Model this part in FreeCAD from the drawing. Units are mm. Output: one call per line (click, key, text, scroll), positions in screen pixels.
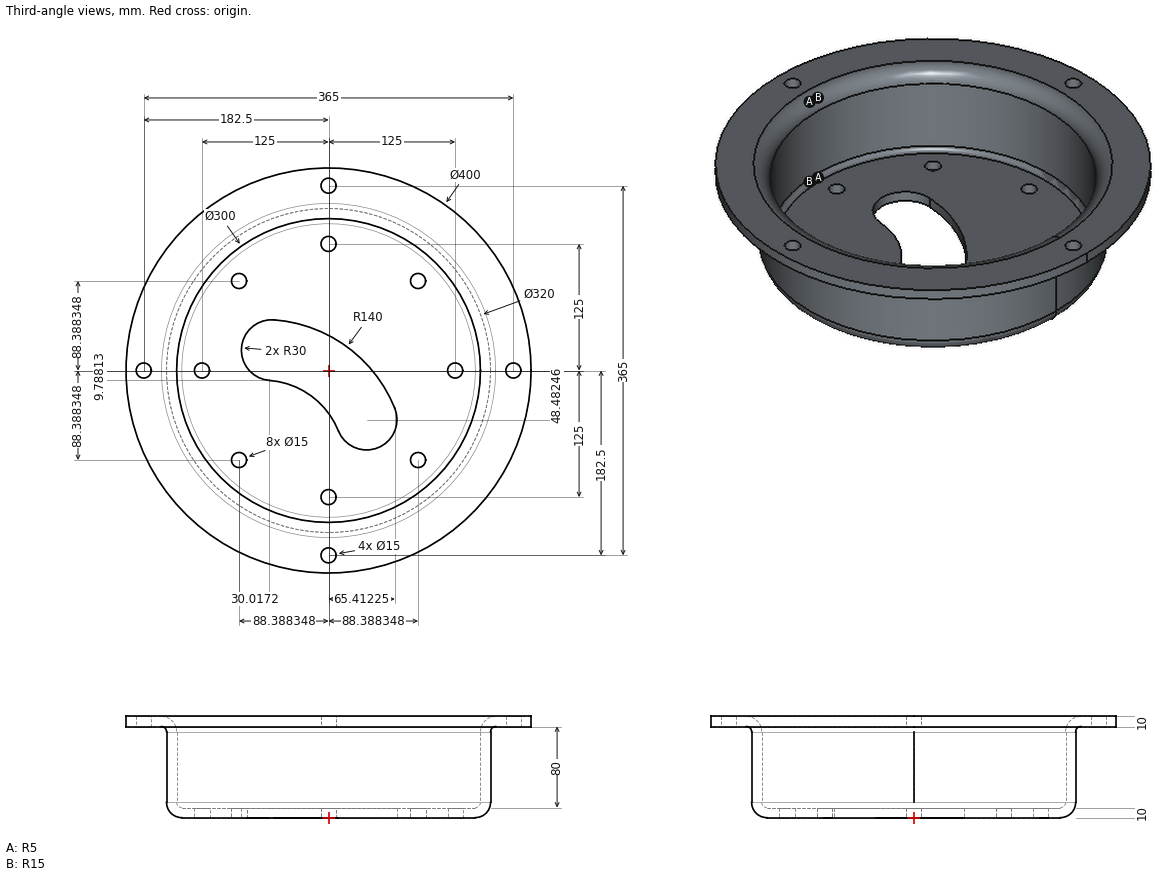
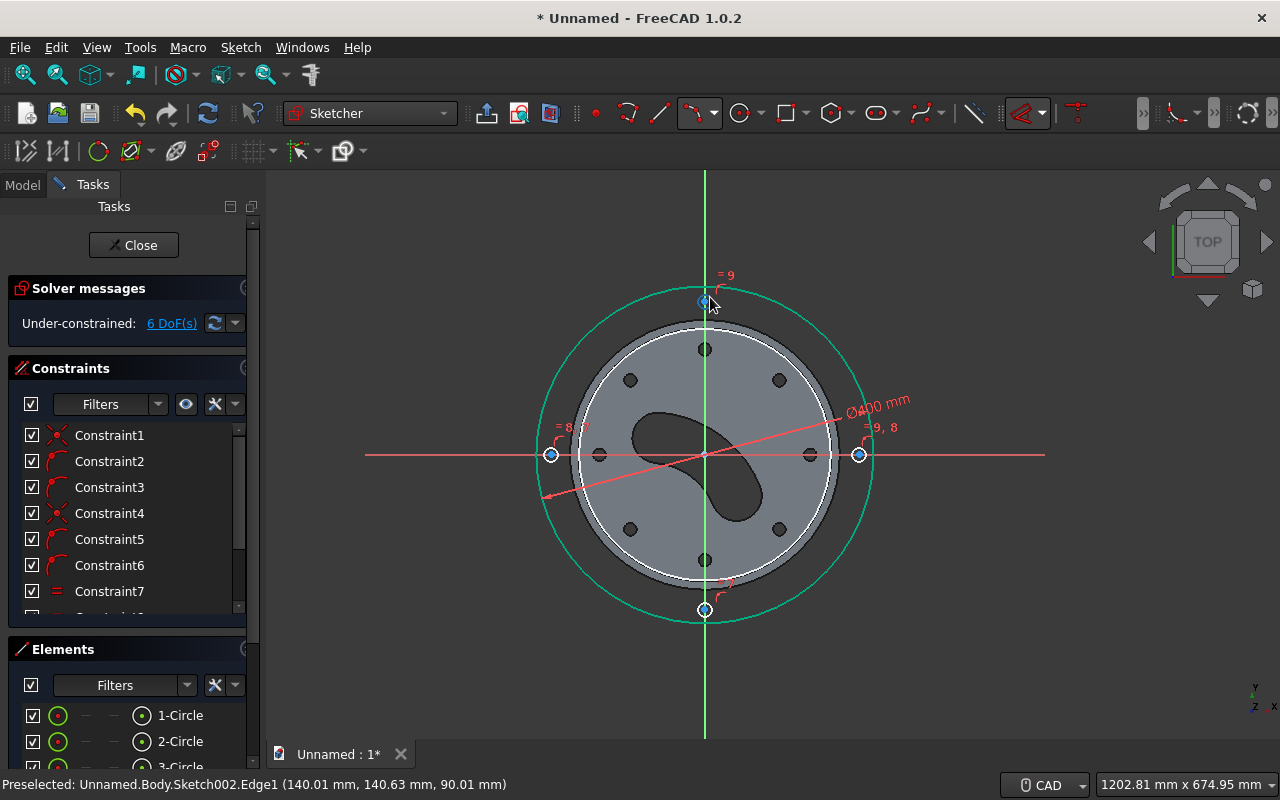
scroll(710, 605, up, 6)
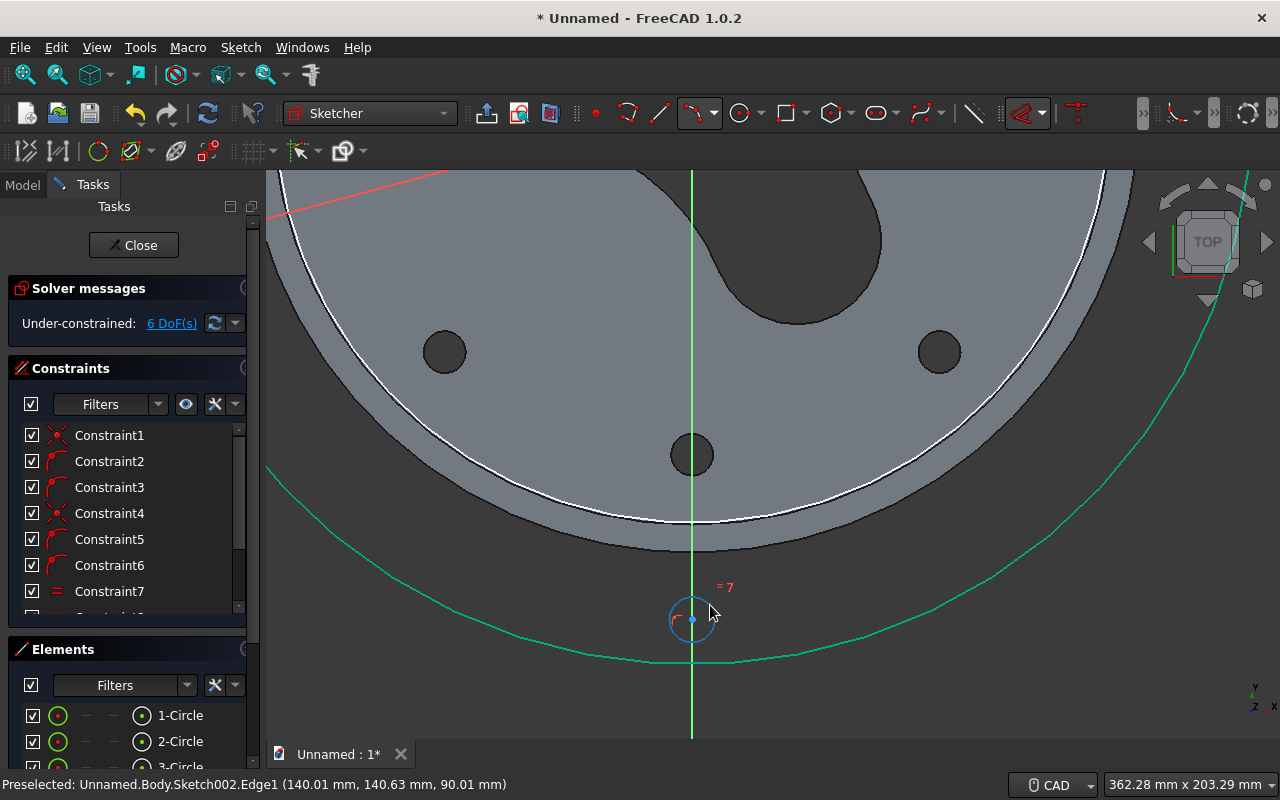
click(708, 604)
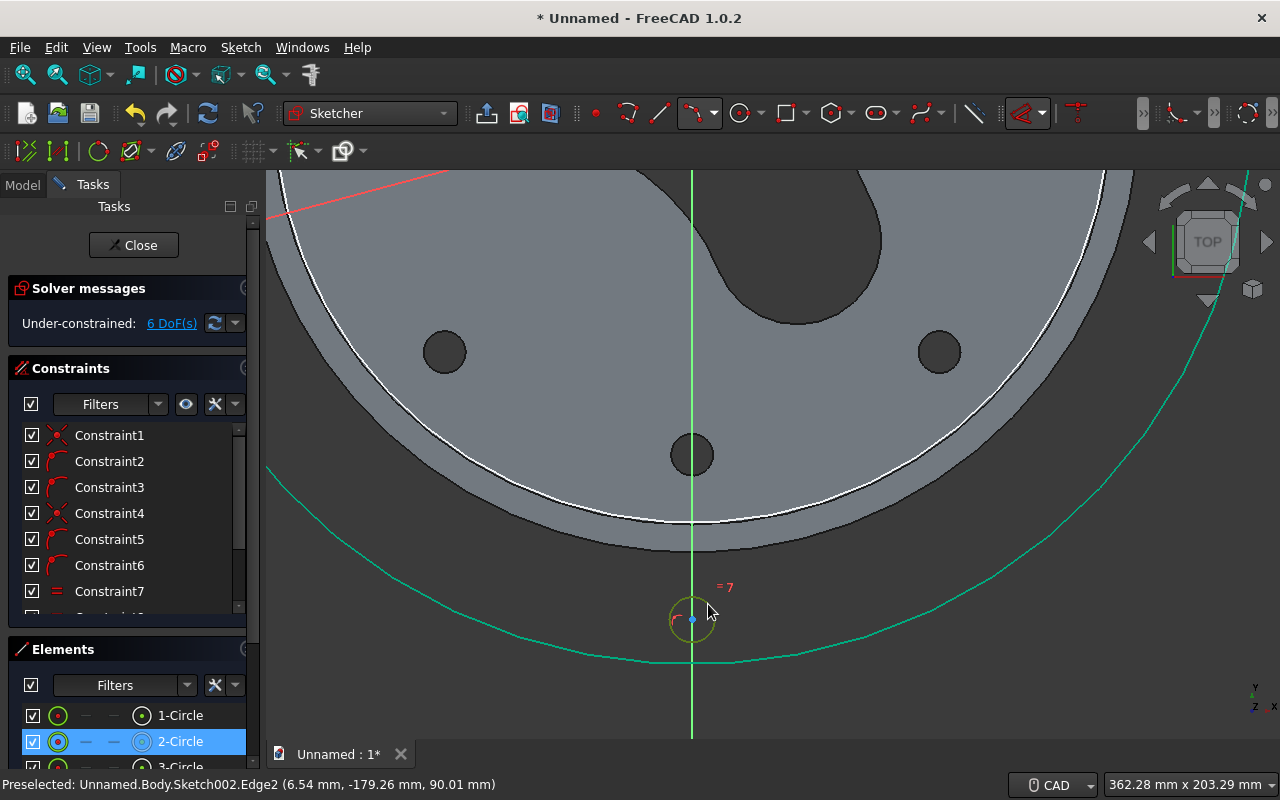
click(1044, 114)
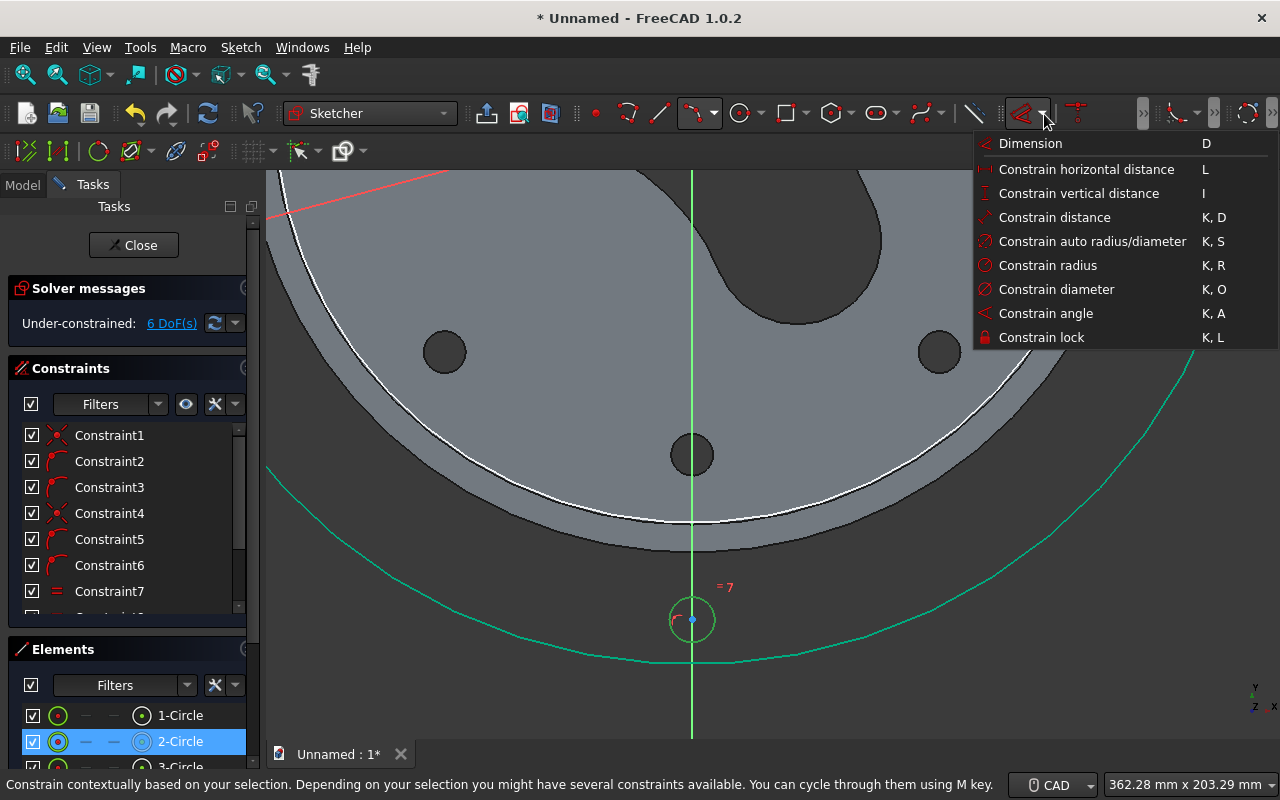
click(1126, 289)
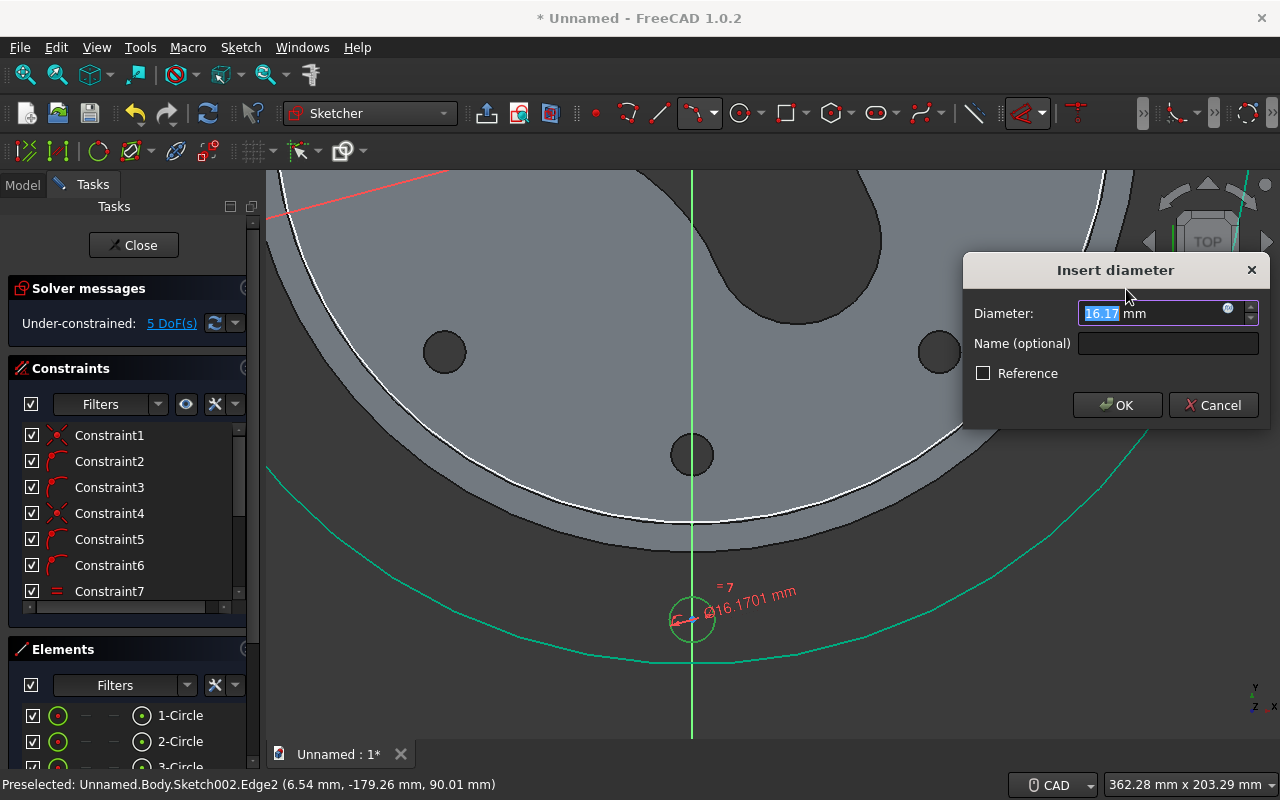
text(15)
key(Return)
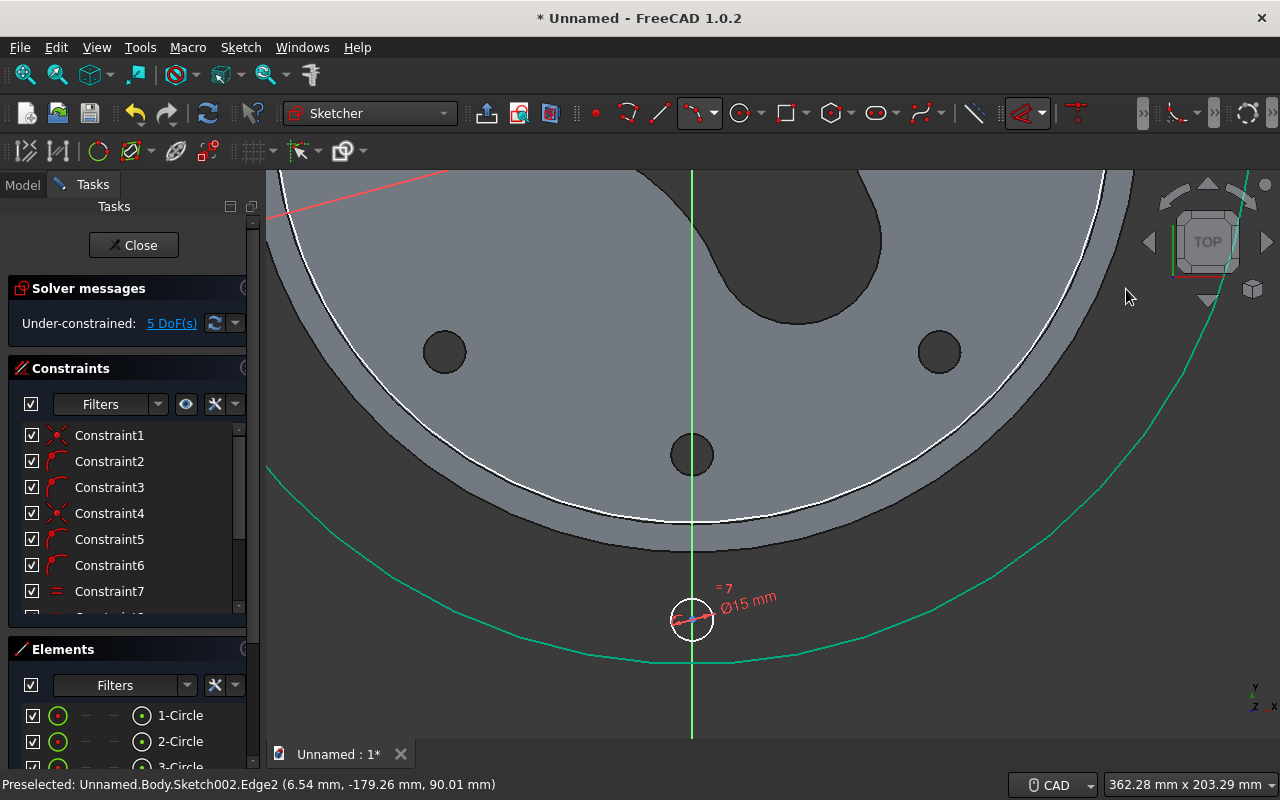
click(398, 401)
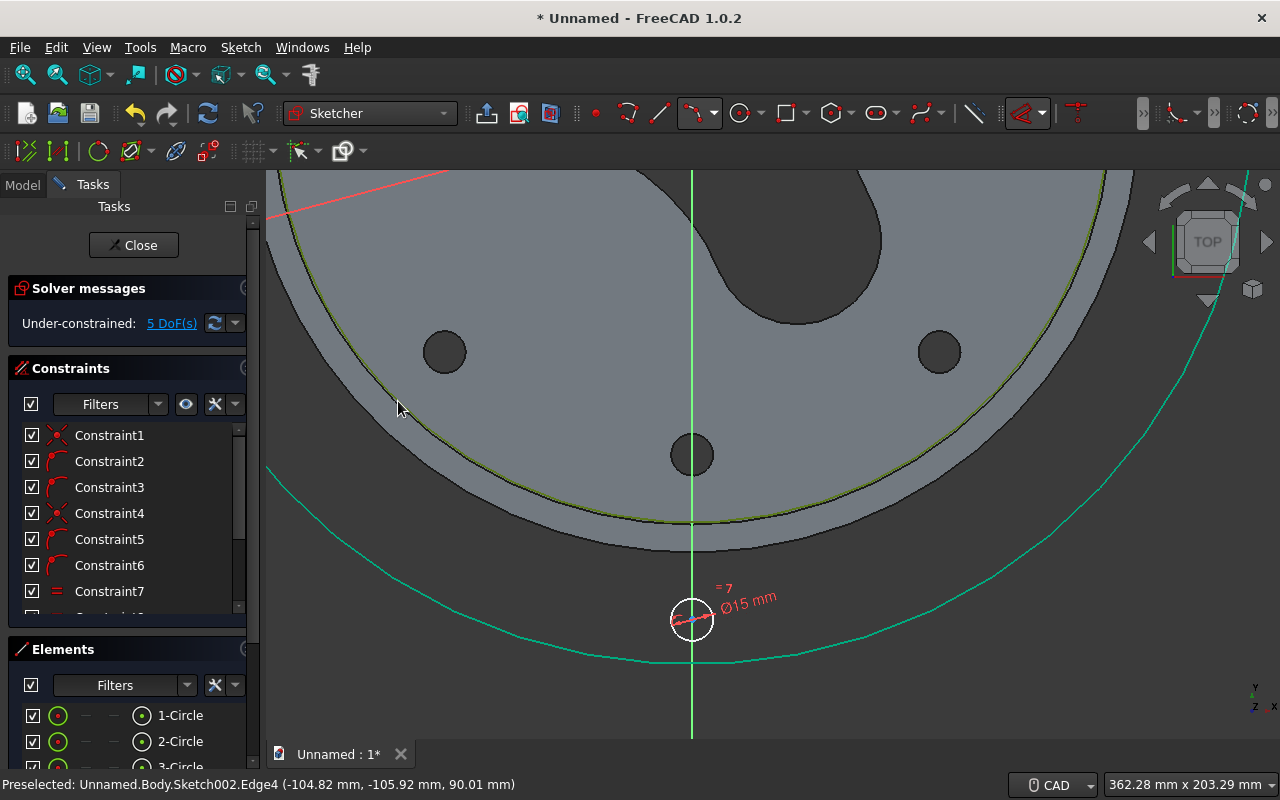
key(k)
key(o)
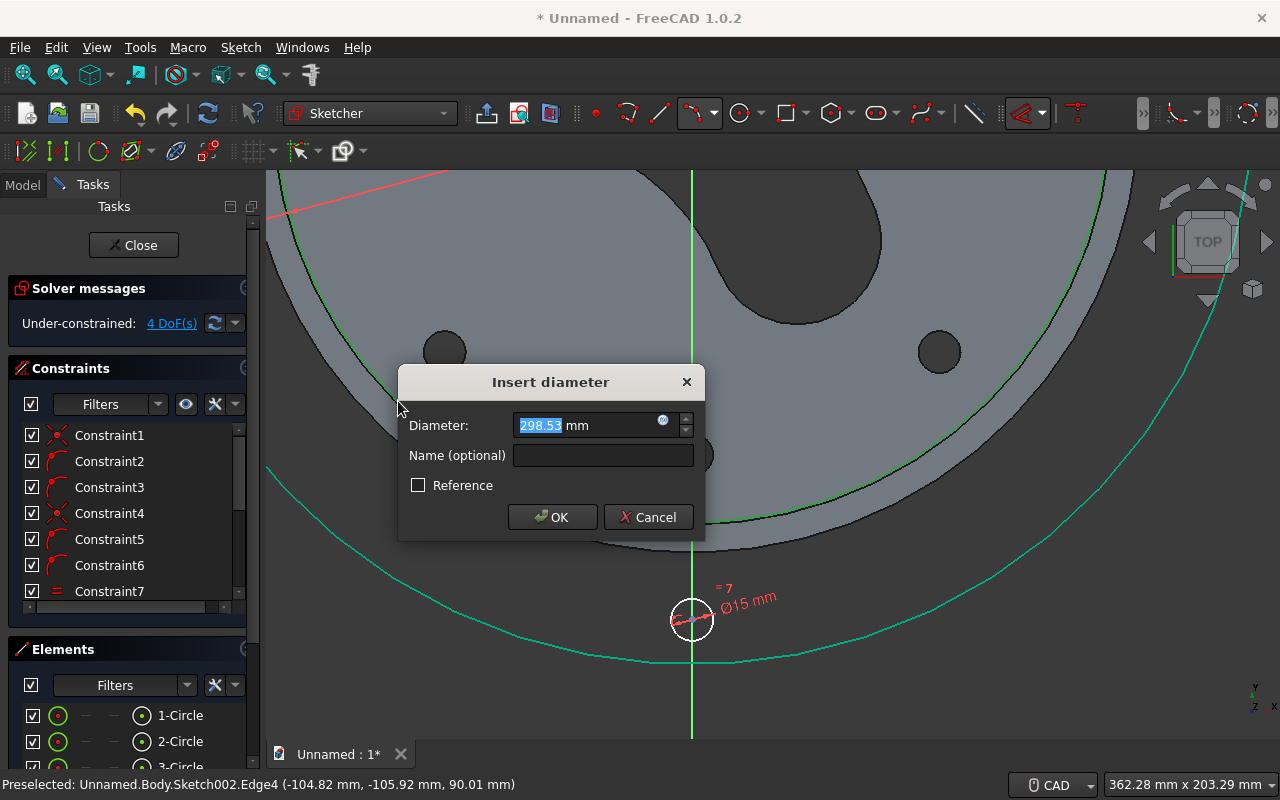
text(300)
key(Return)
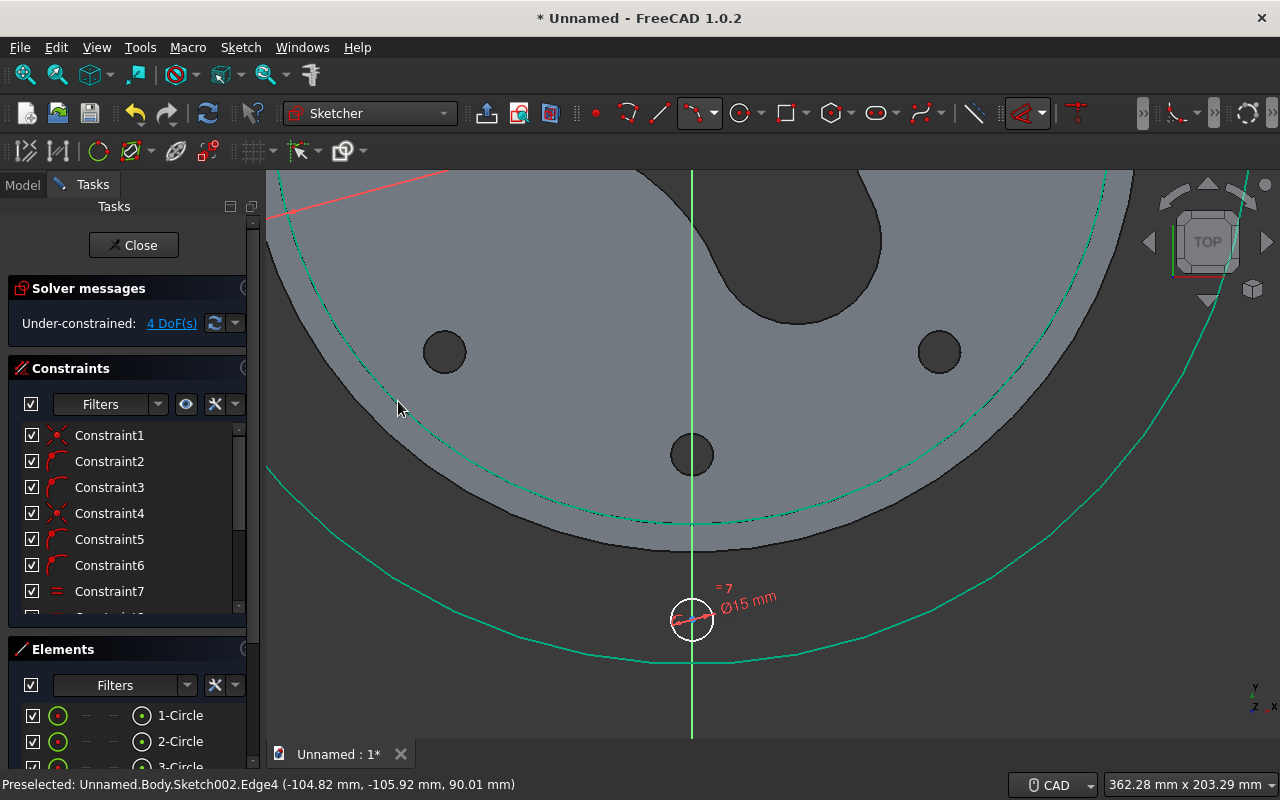
scroll(710, 605, down, 6)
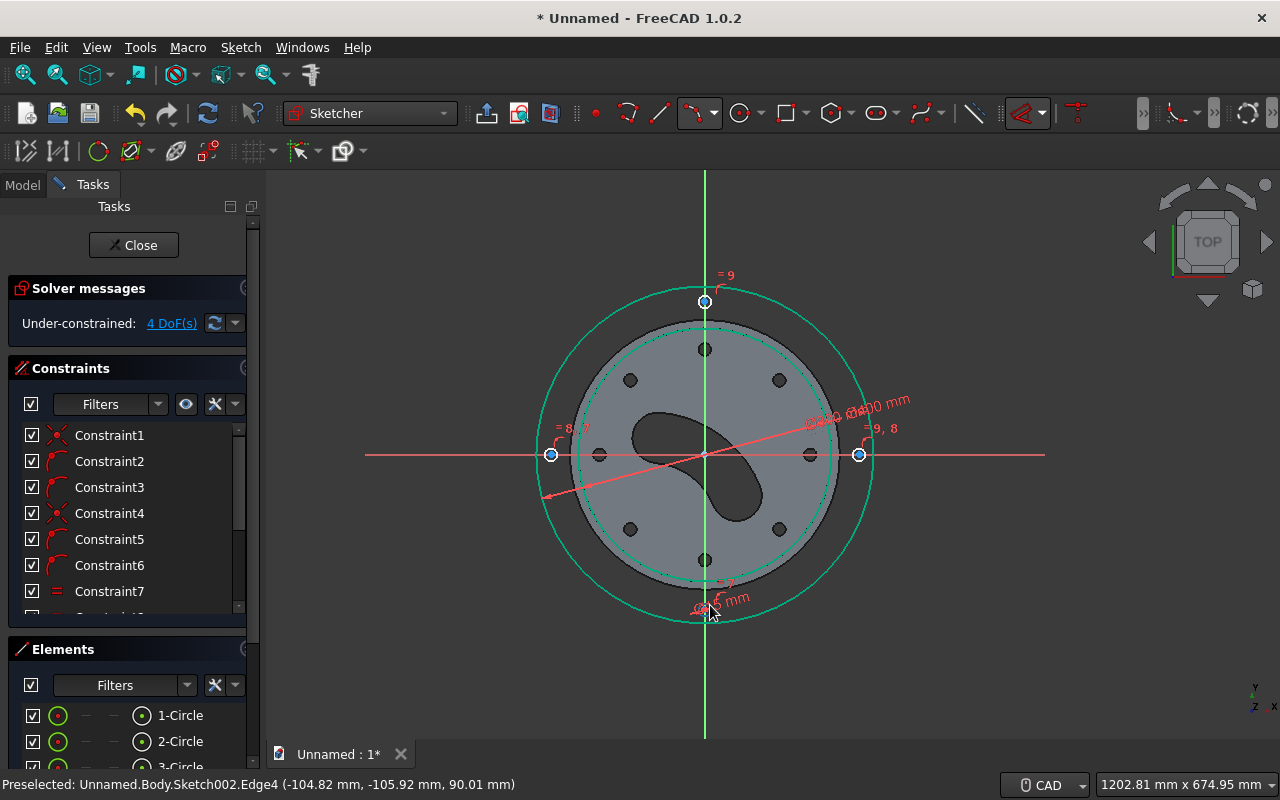
click(551, 455)